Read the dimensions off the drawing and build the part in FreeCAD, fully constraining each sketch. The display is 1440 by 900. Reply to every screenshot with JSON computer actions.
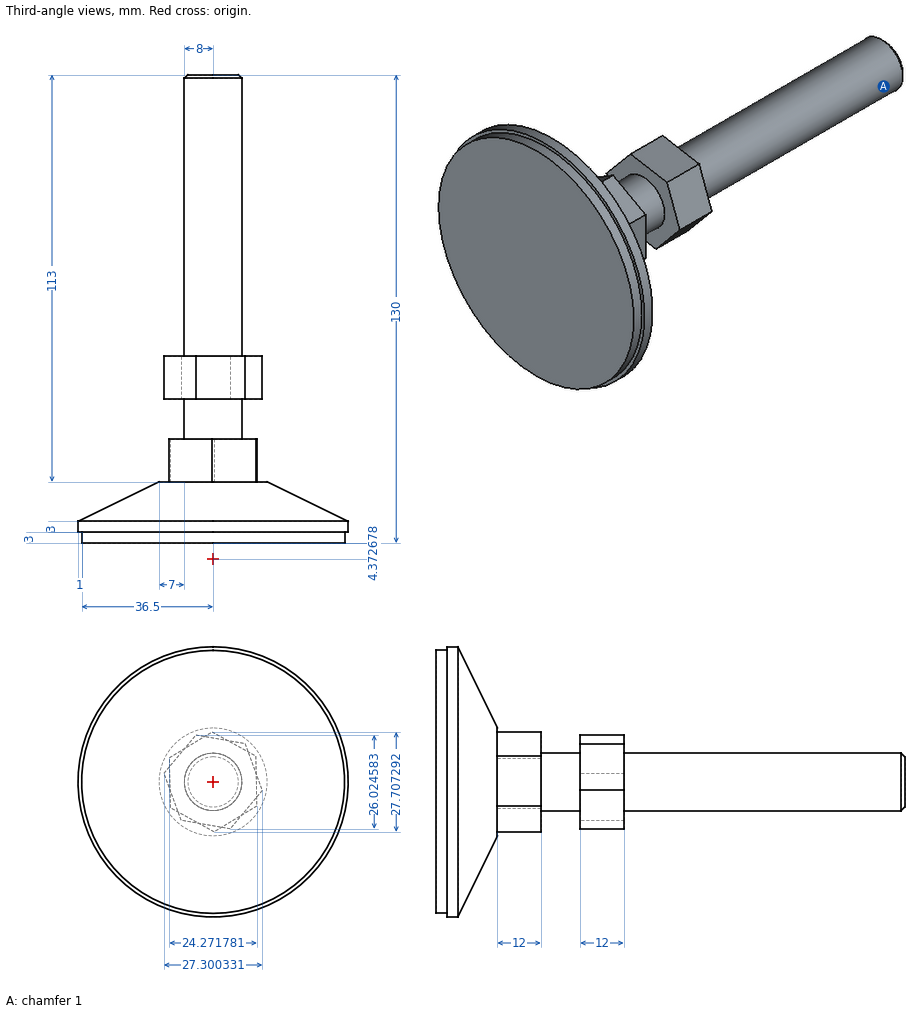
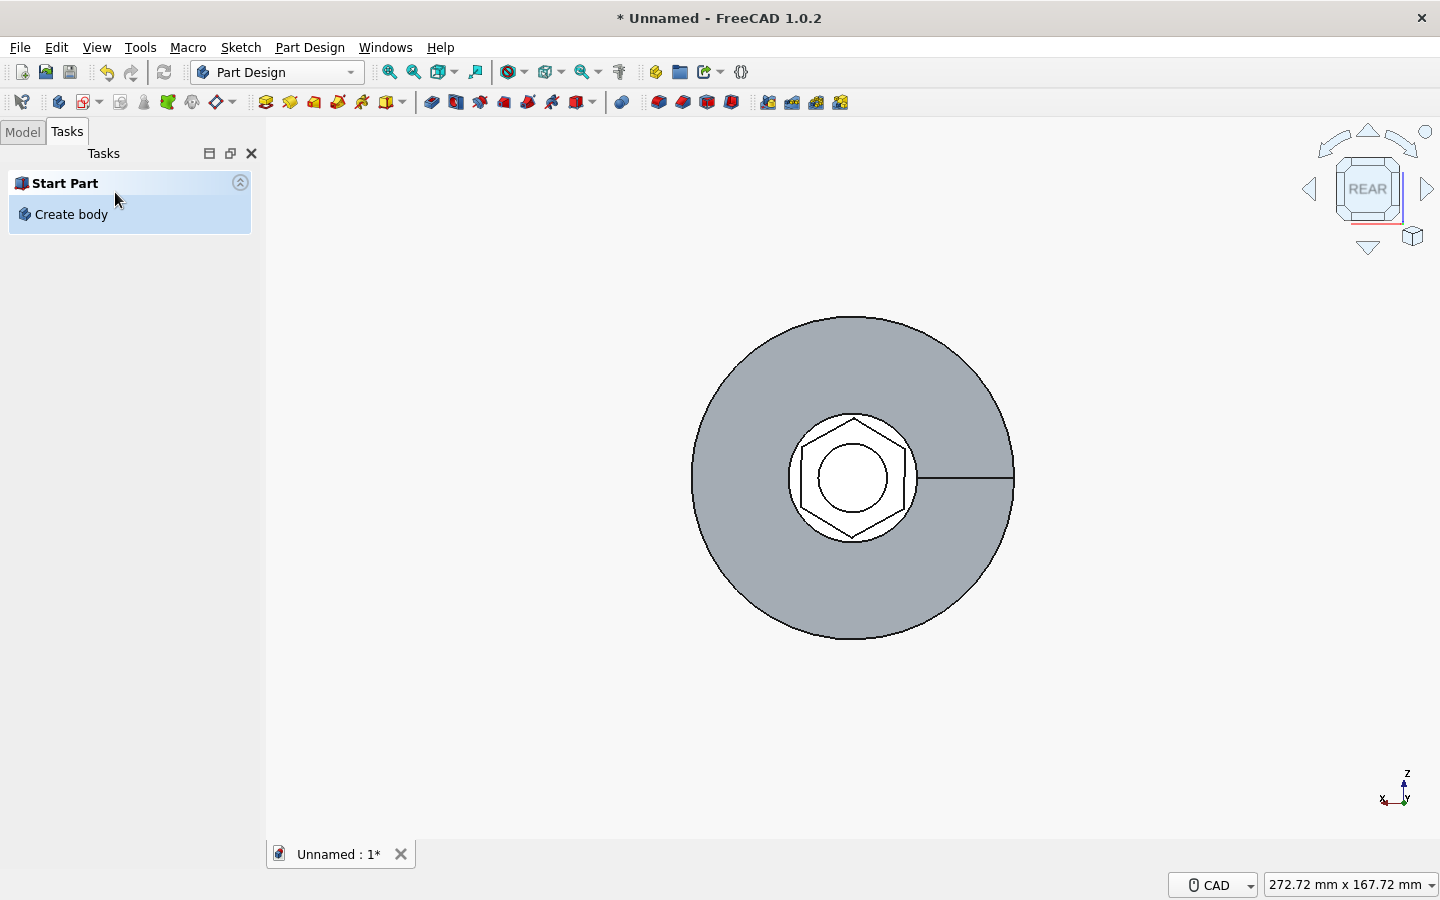
{"action": "left_click", "coordinate": [390, 72]}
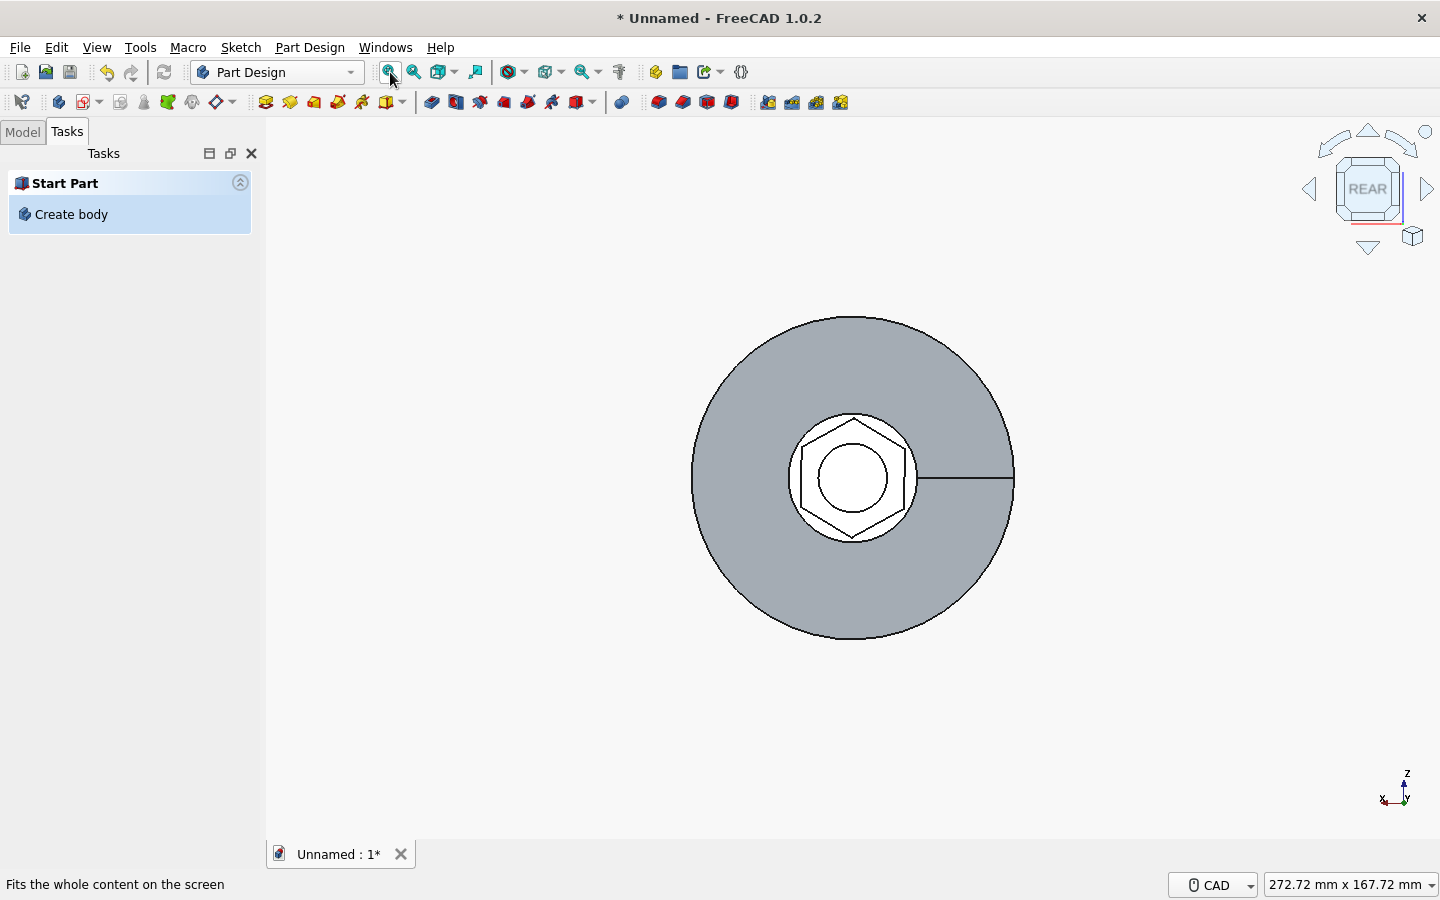
{"action": "left_click", "coordinate": [23, 131]}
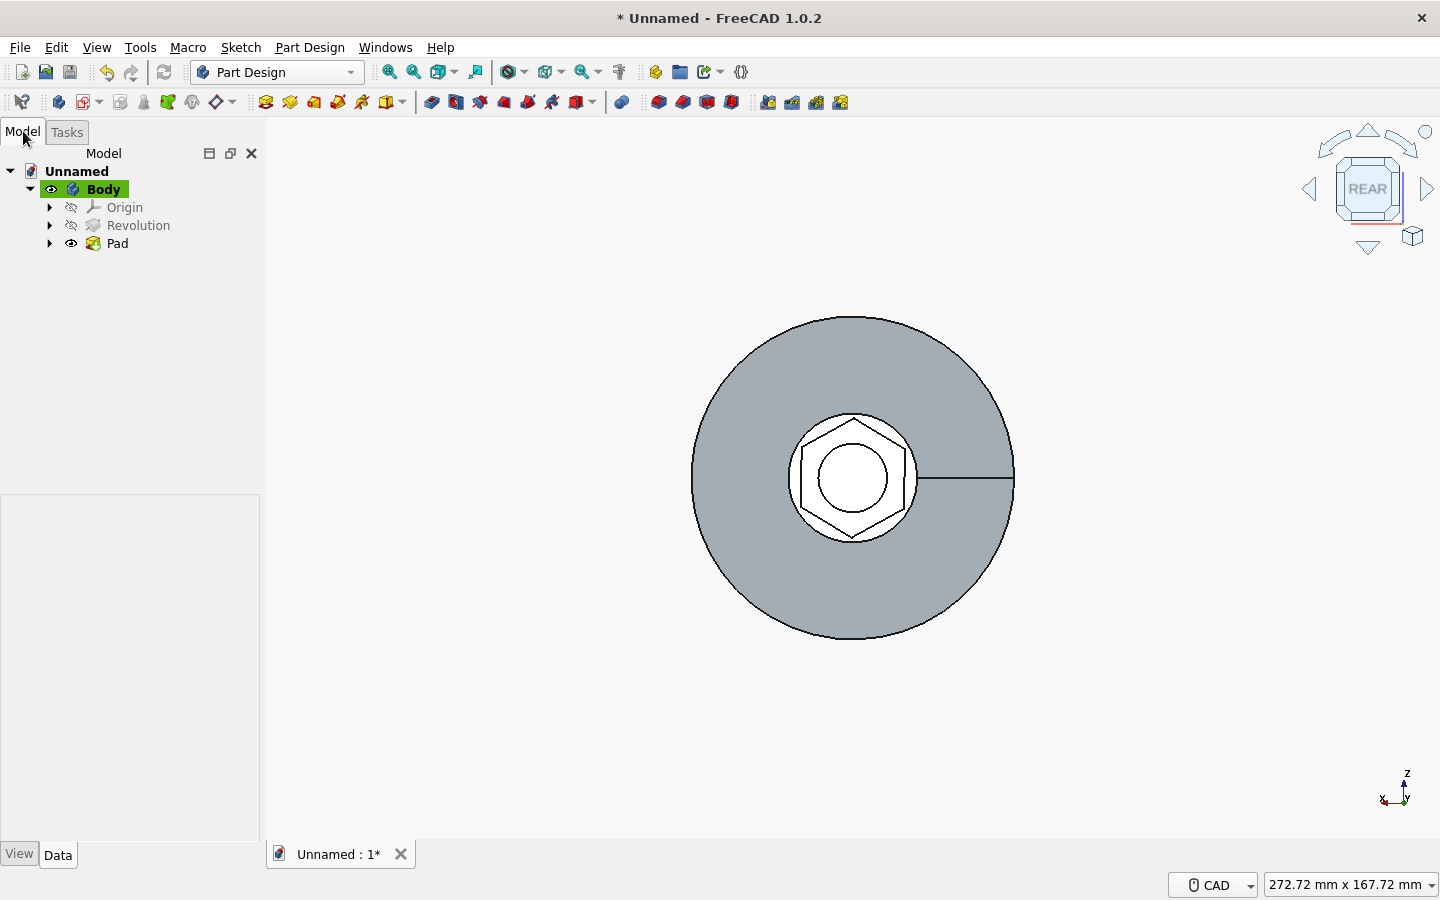
{"action": "left_click", "coordinate": [50, 207]}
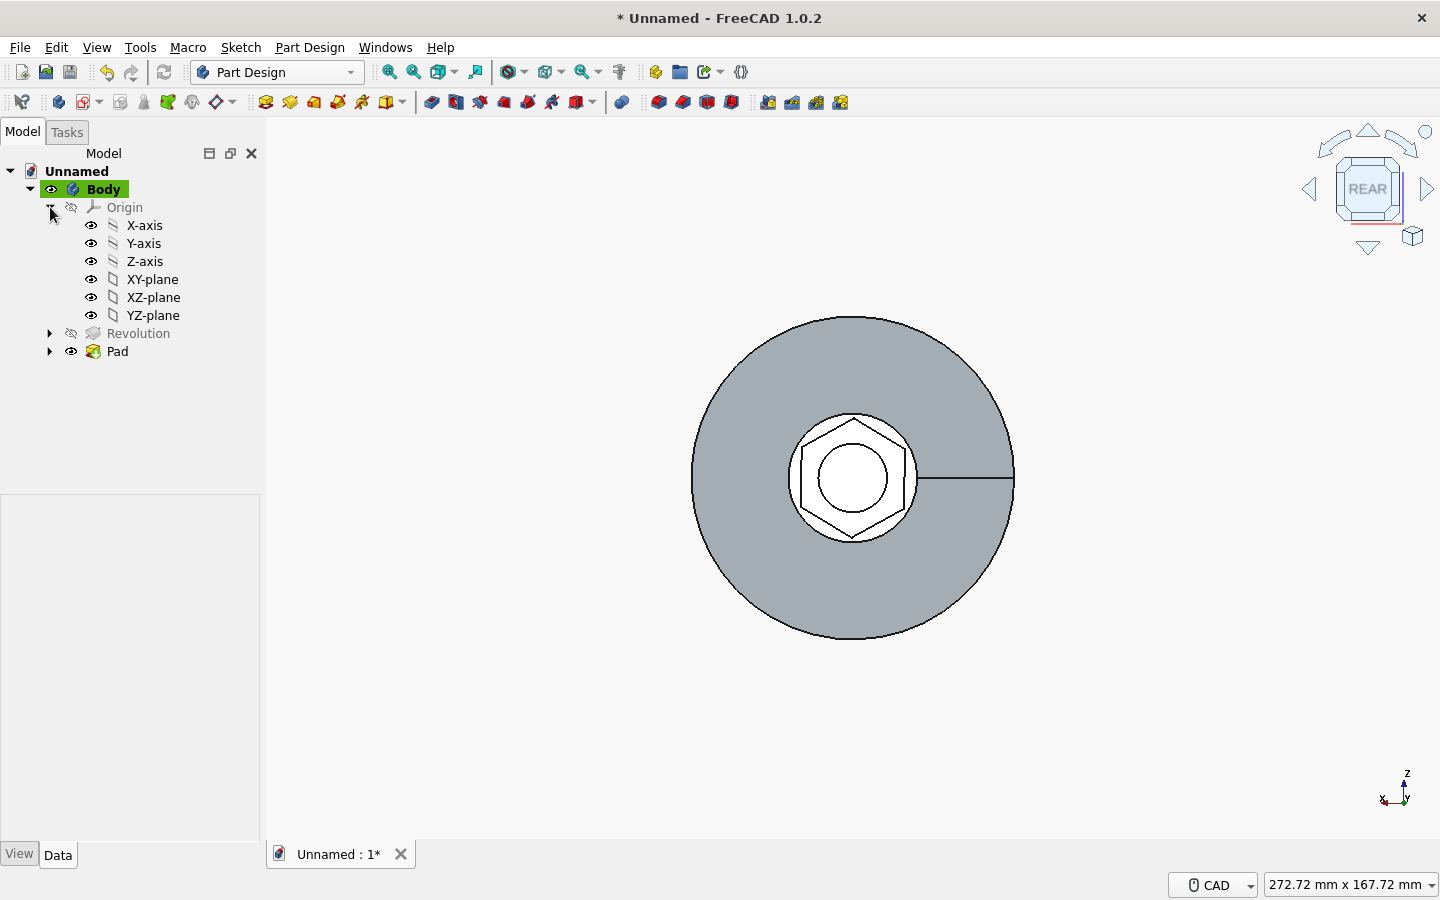
{"action": "left_click", "coordinate": [136, 297]}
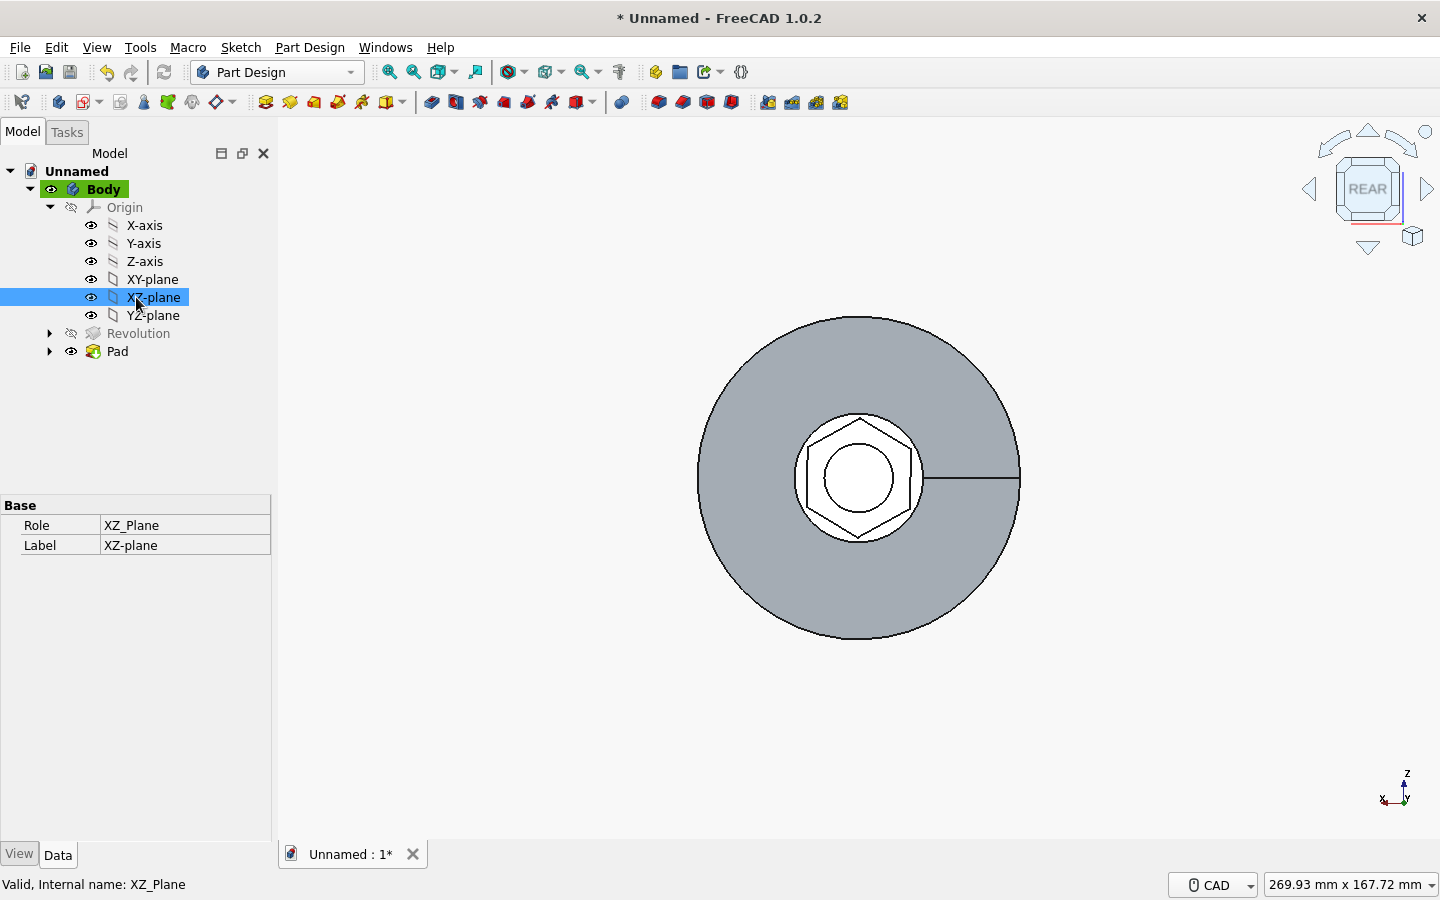
{"action": "left_click", "coordinate": [216, 102]}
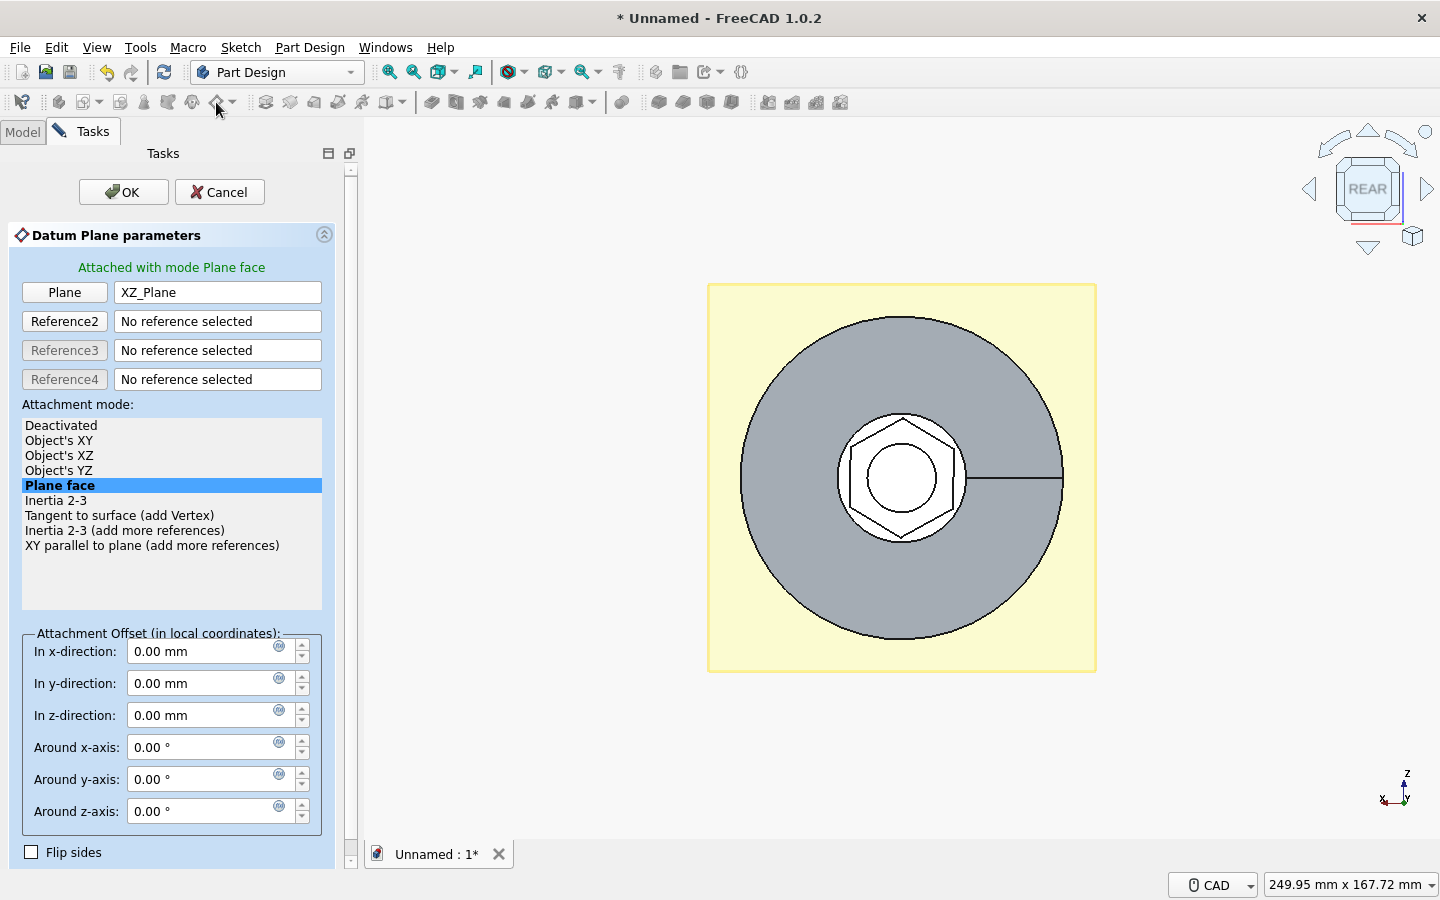
{"action": "triple_click", "coordinate": [210, 715]}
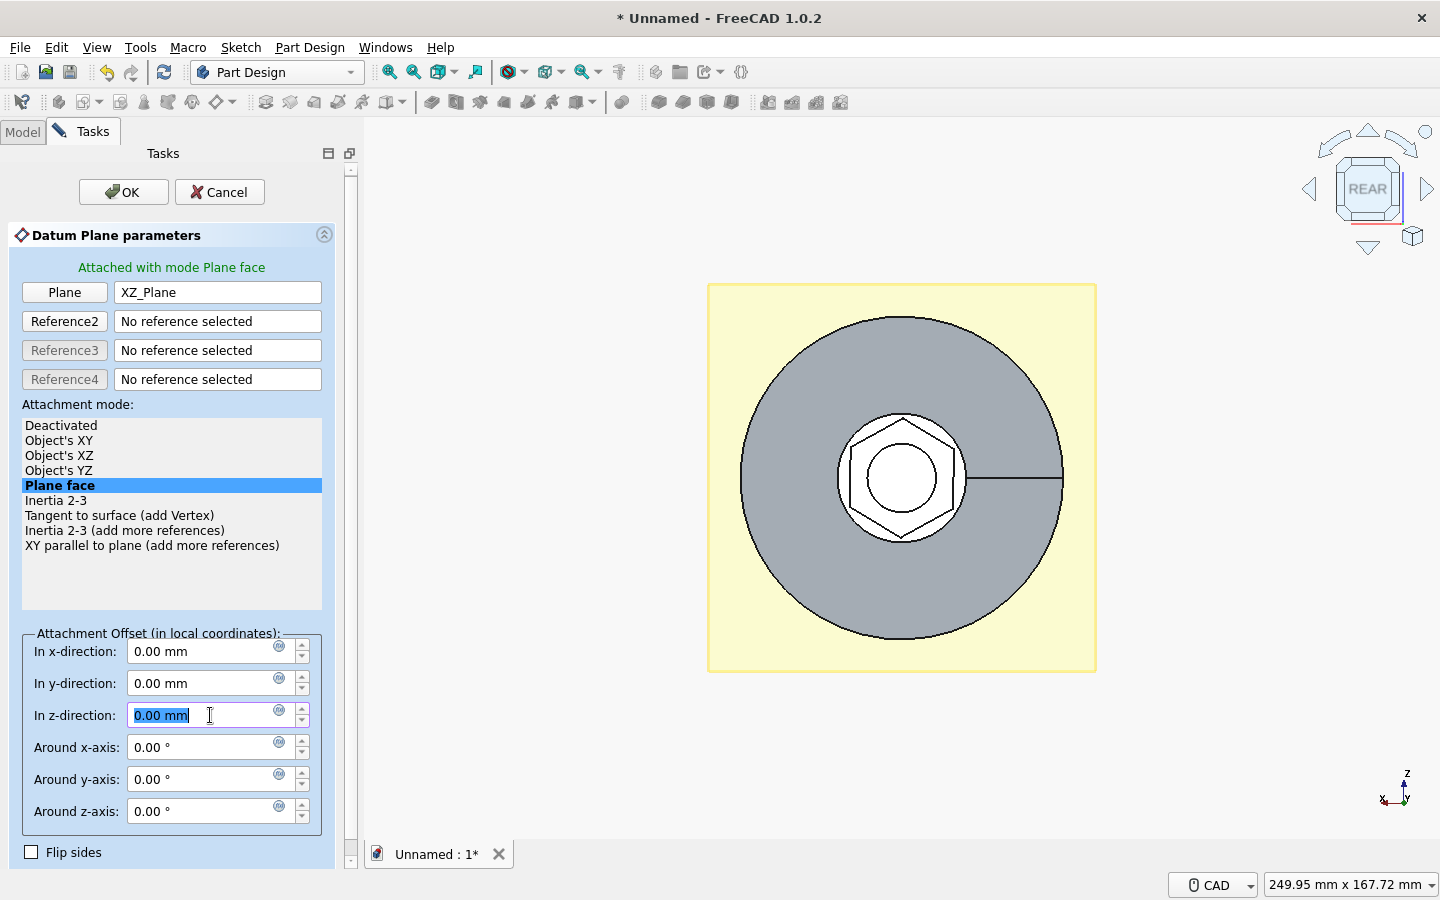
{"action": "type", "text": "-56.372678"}
{"action": "key", "text": "Tab"}